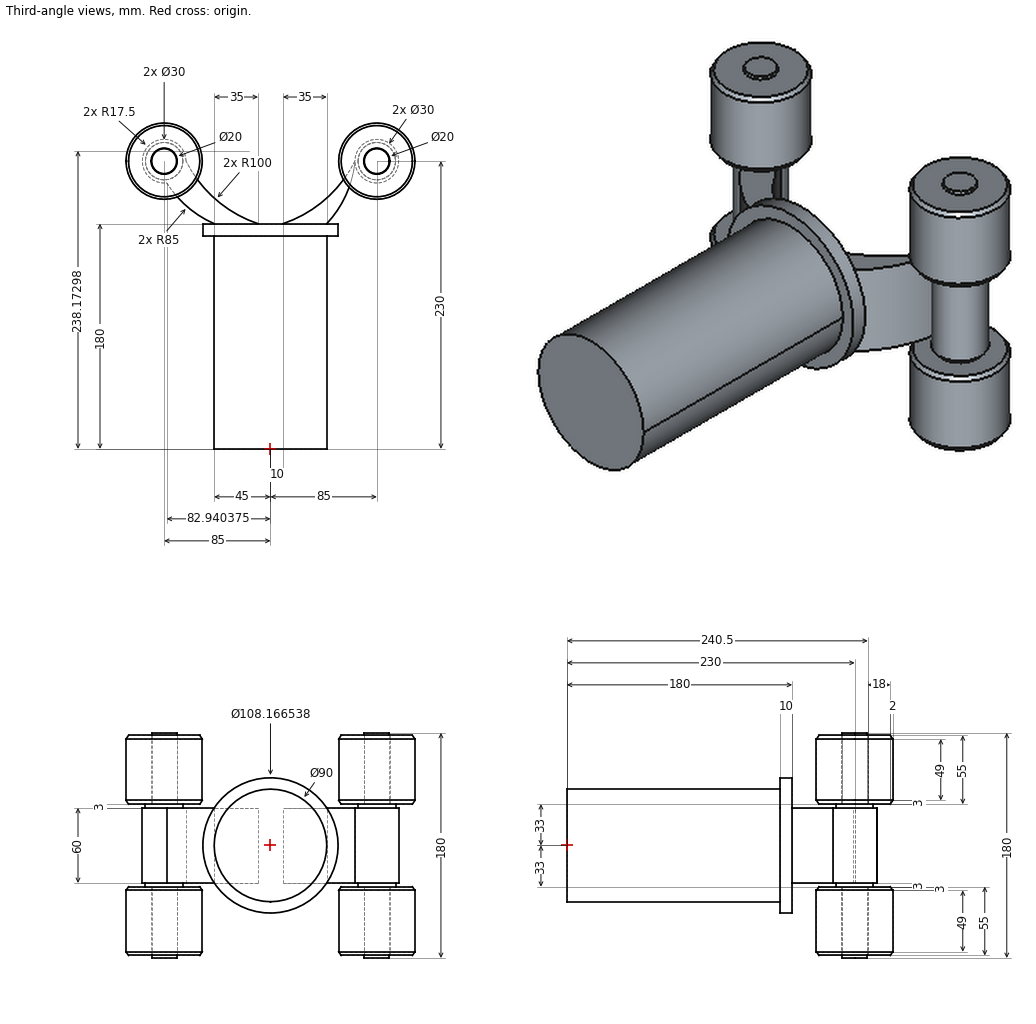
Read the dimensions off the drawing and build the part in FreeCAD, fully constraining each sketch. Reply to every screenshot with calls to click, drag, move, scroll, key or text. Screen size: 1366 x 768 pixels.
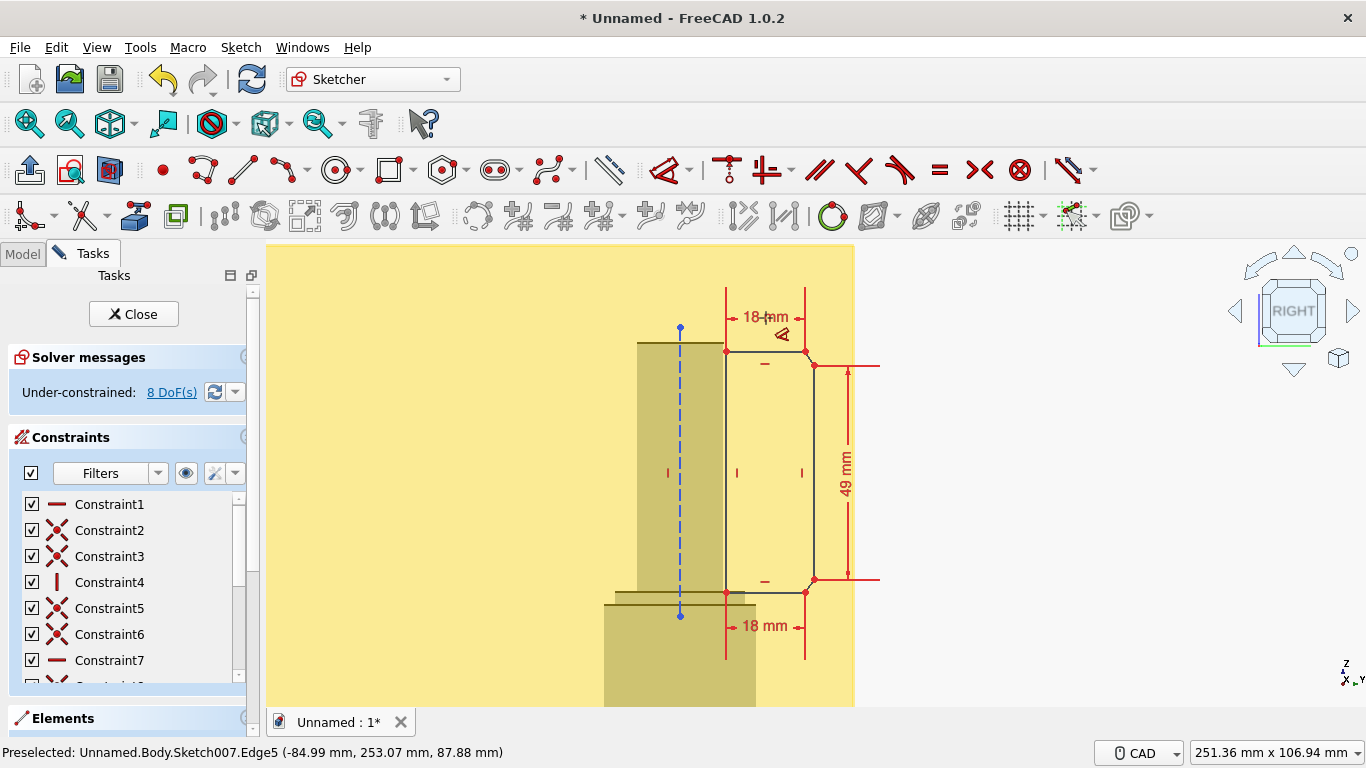
click(726, 424)
click(760, 472)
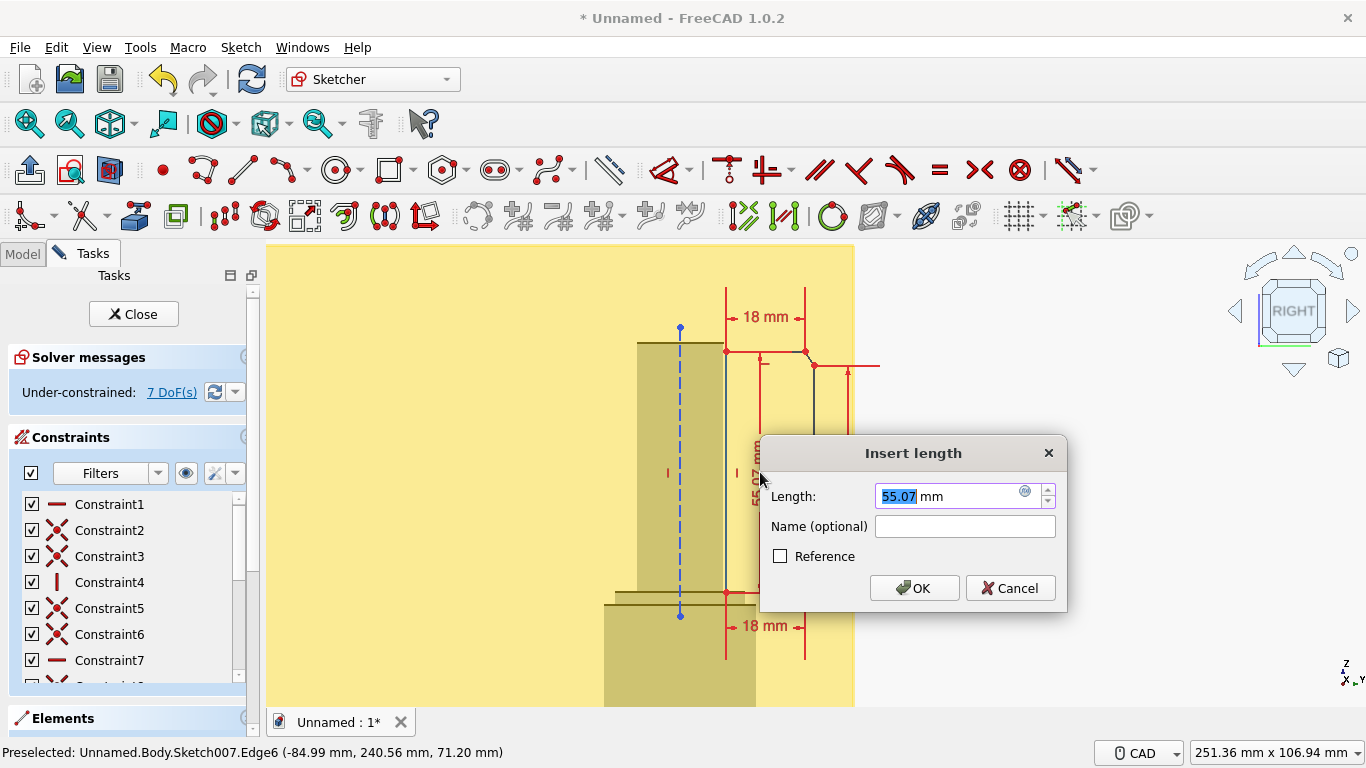
text(55)
key(Return)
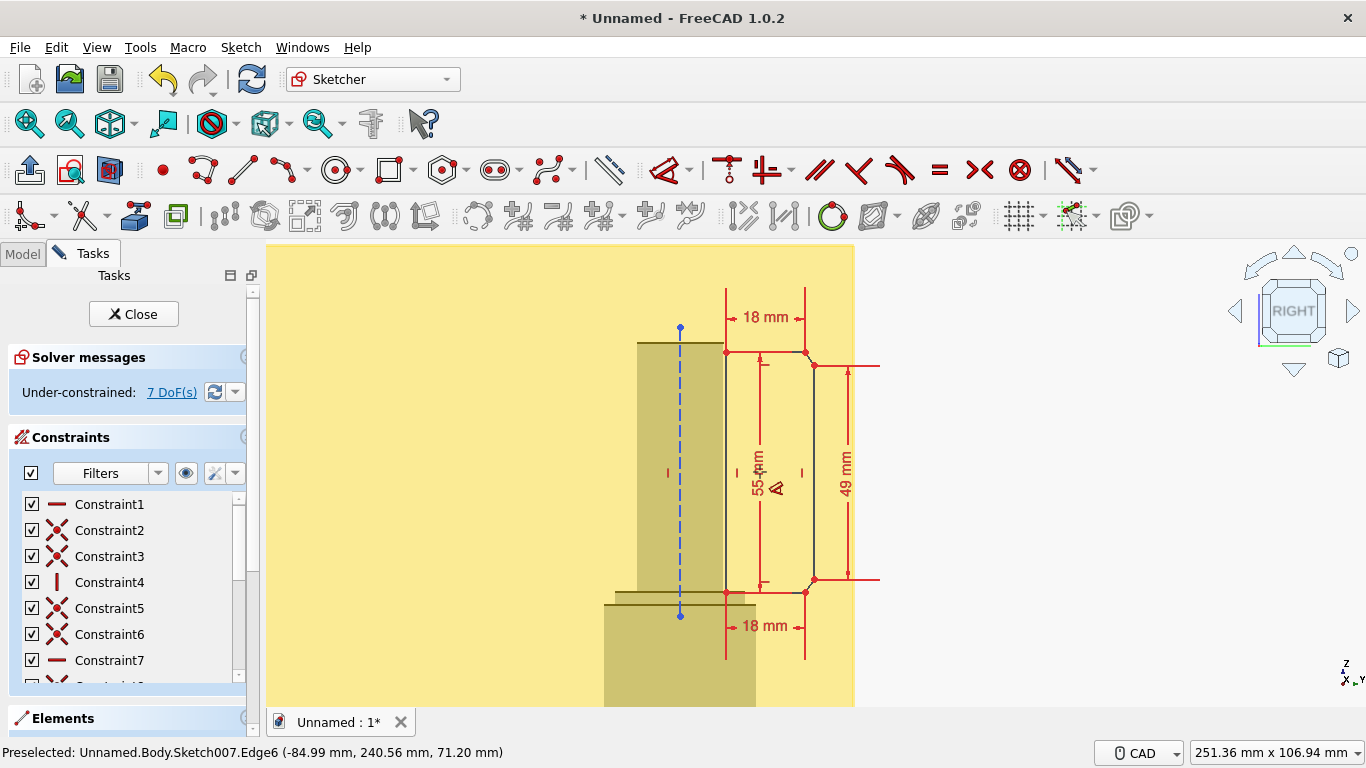
scroll(810, 587, up, 8)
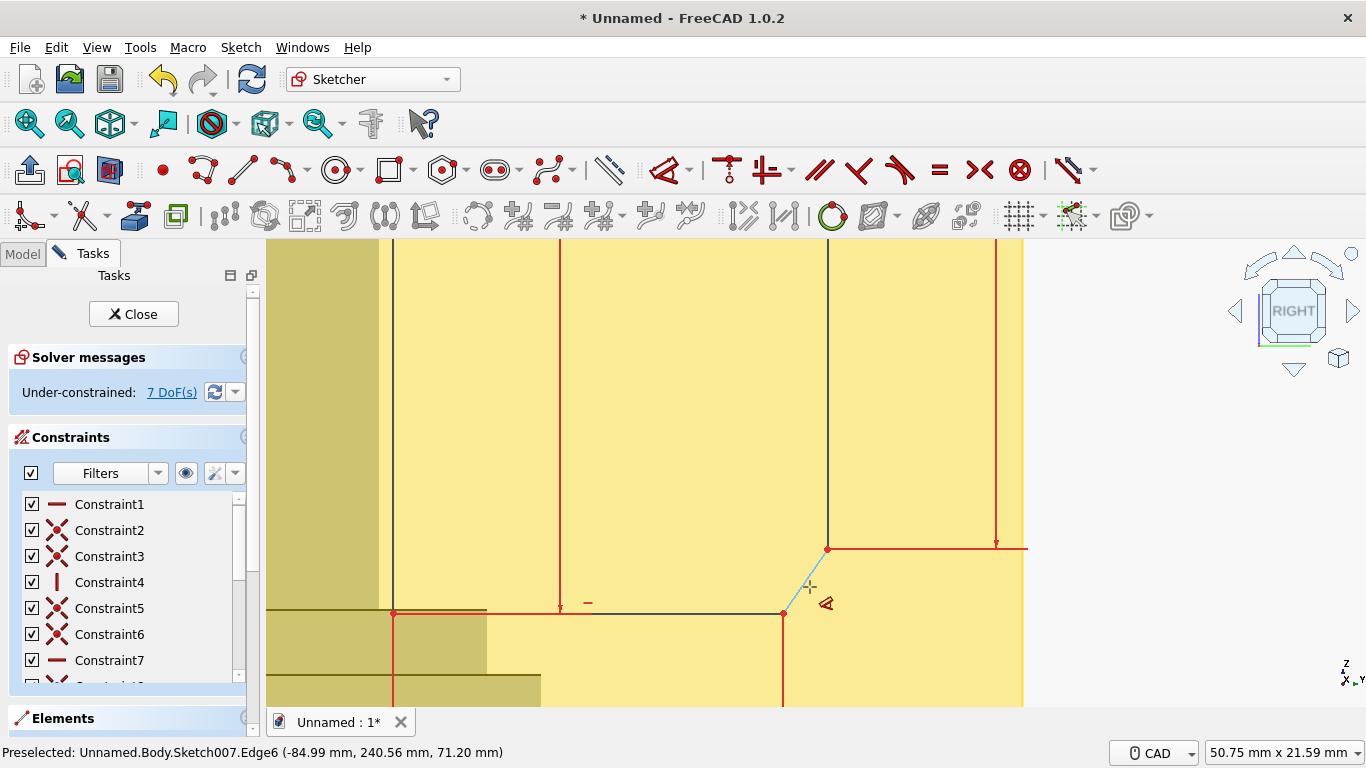
click(806, 582)
click(806, 648)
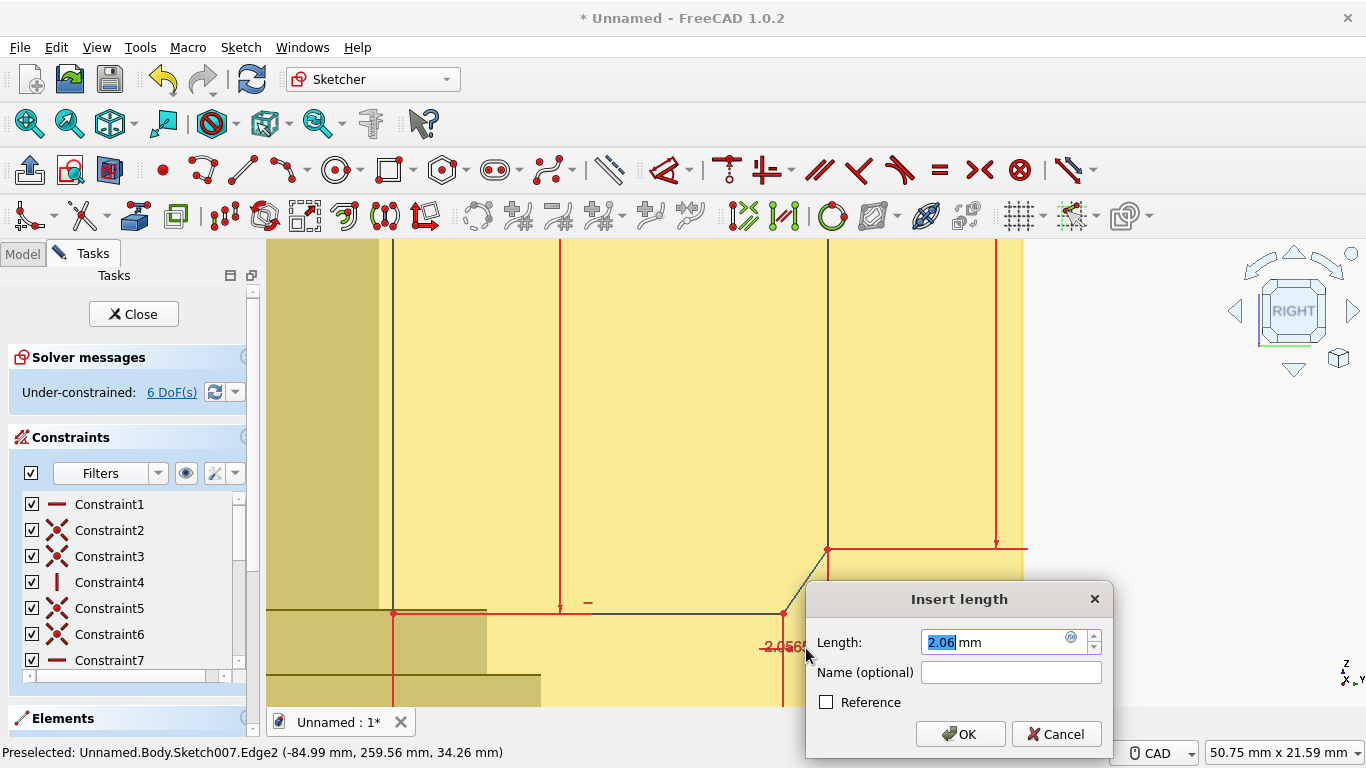
text(2)
key(Return)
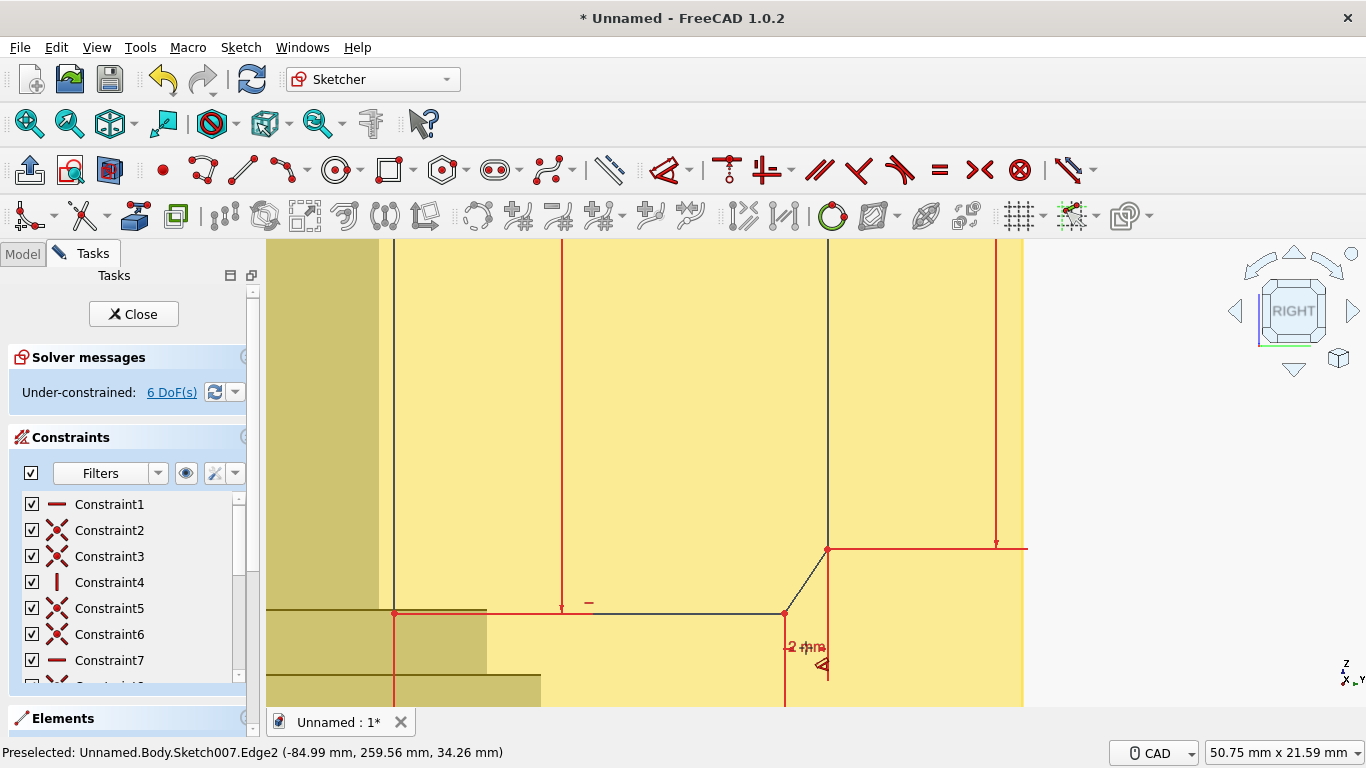
click(798, 594)
click(862, 582)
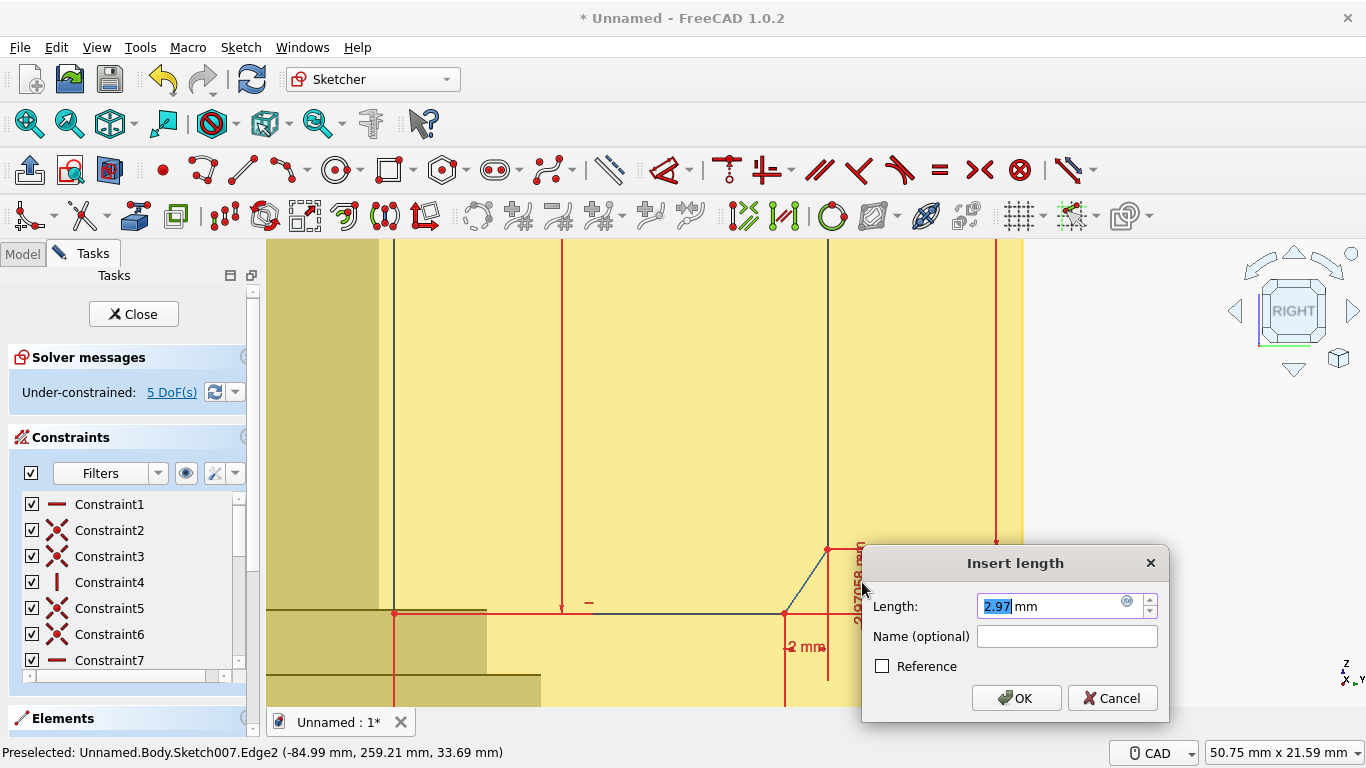
text(3)
key(Return)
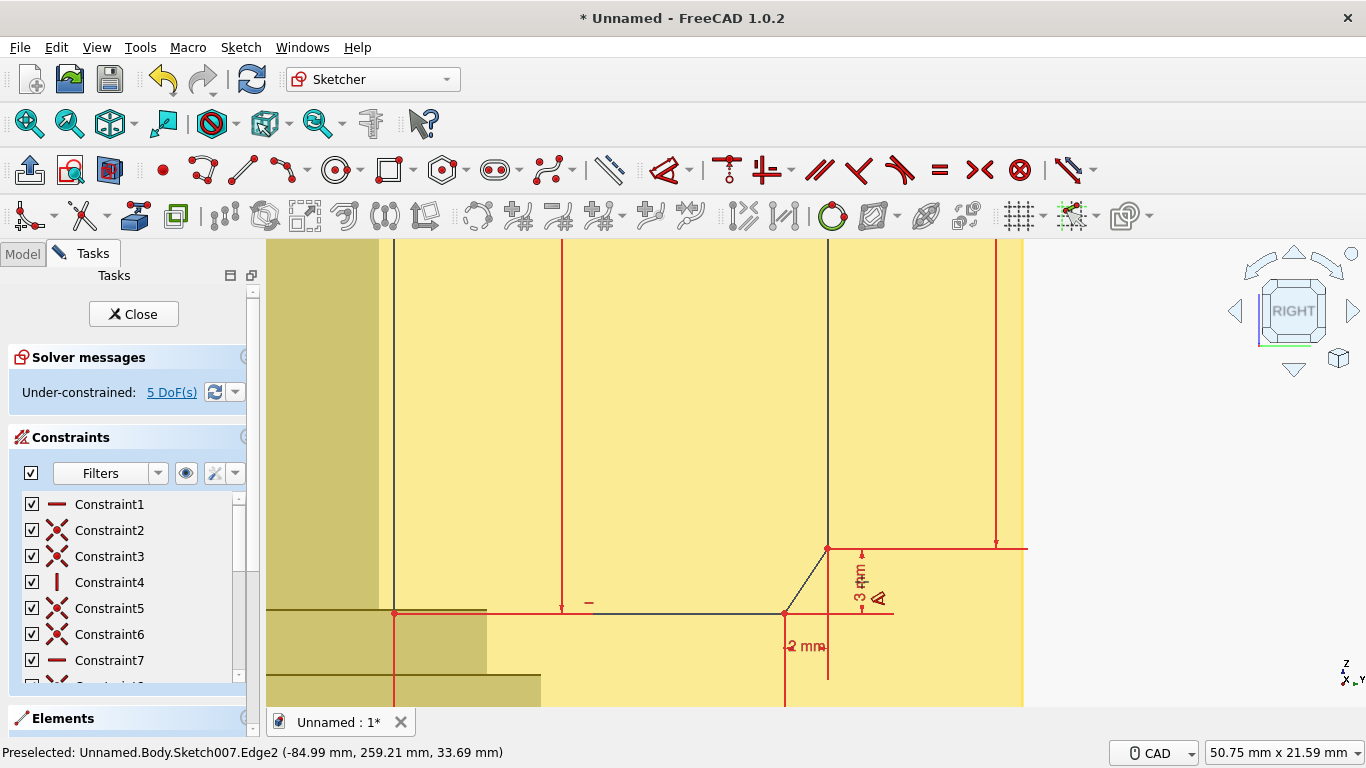
scroll(811, 589, down, 8)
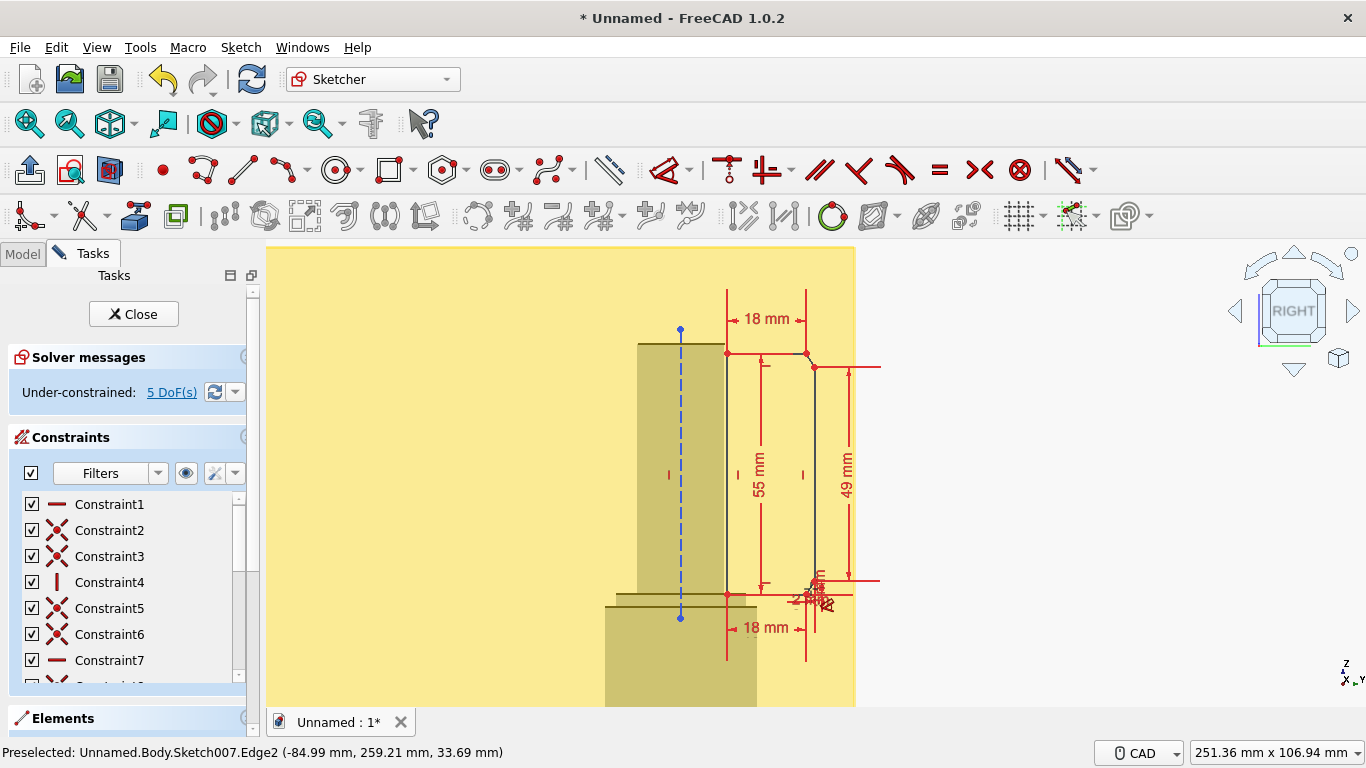
click(727, 595)
click(761, 656)